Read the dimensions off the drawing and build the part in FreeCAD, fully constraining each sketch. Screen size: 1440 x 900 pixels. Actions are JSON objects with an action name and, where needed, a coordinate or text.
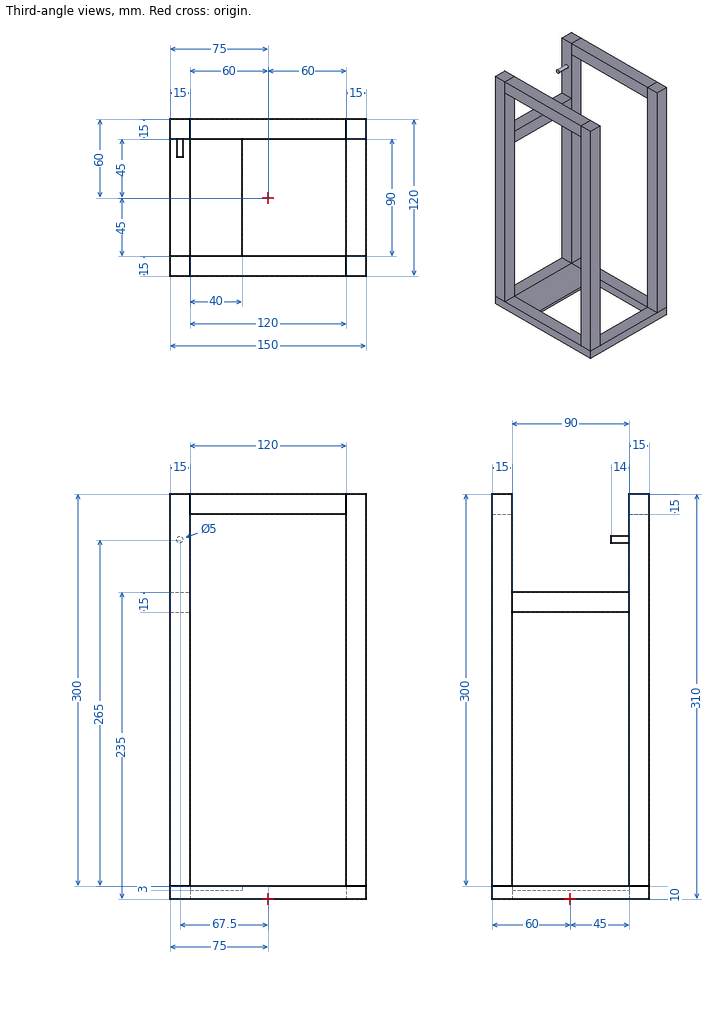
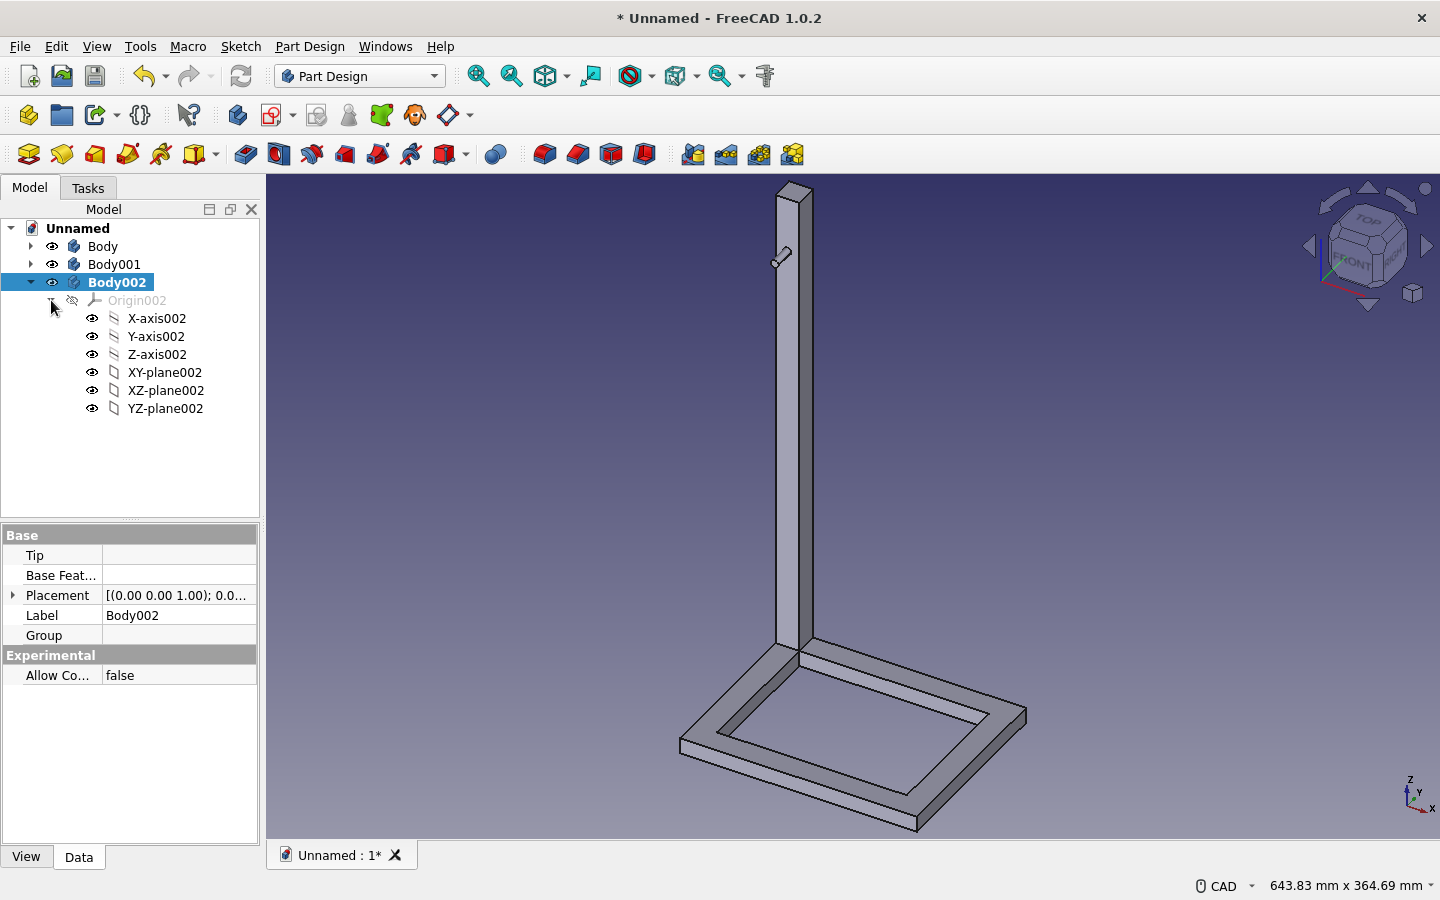
{"action": "left_click", "coordinate": [137, 372]}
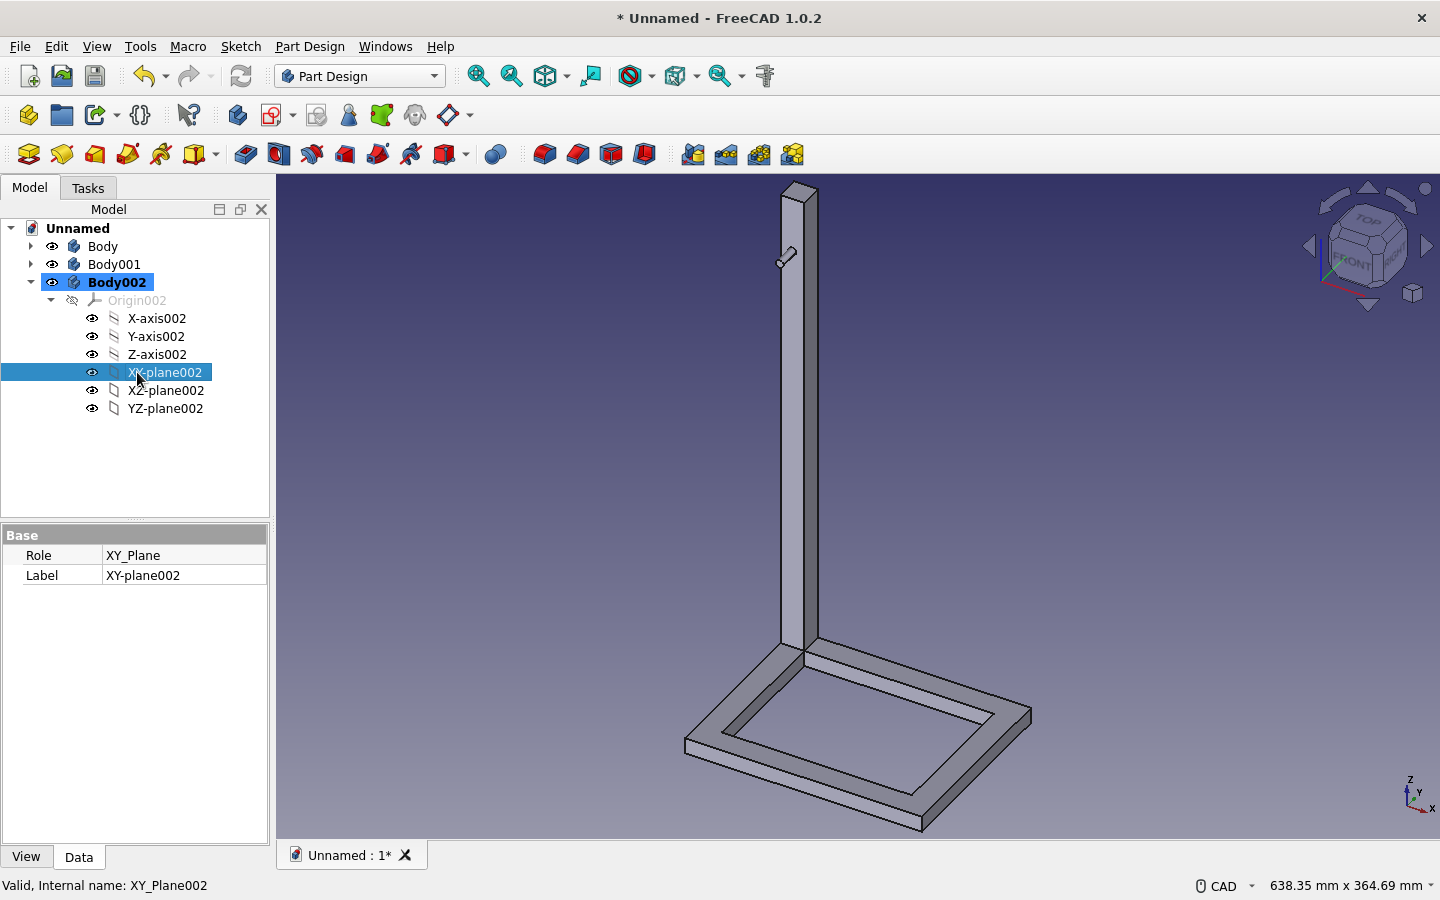
{"action": "left_click", "coordinate": [448, 116]}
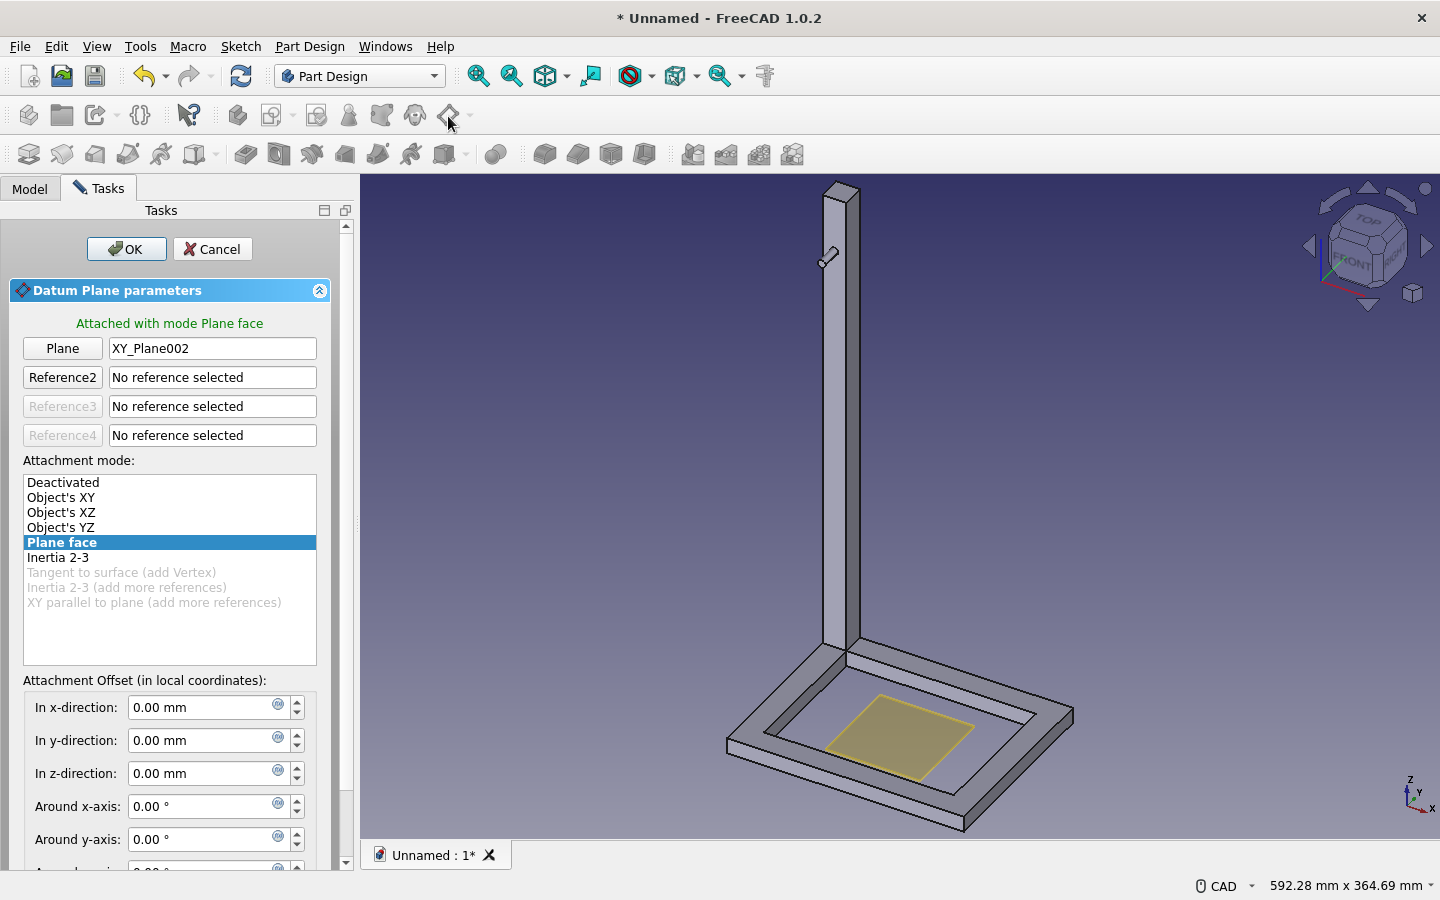
{"action": "triple_click", "coordinate": [210, 774]}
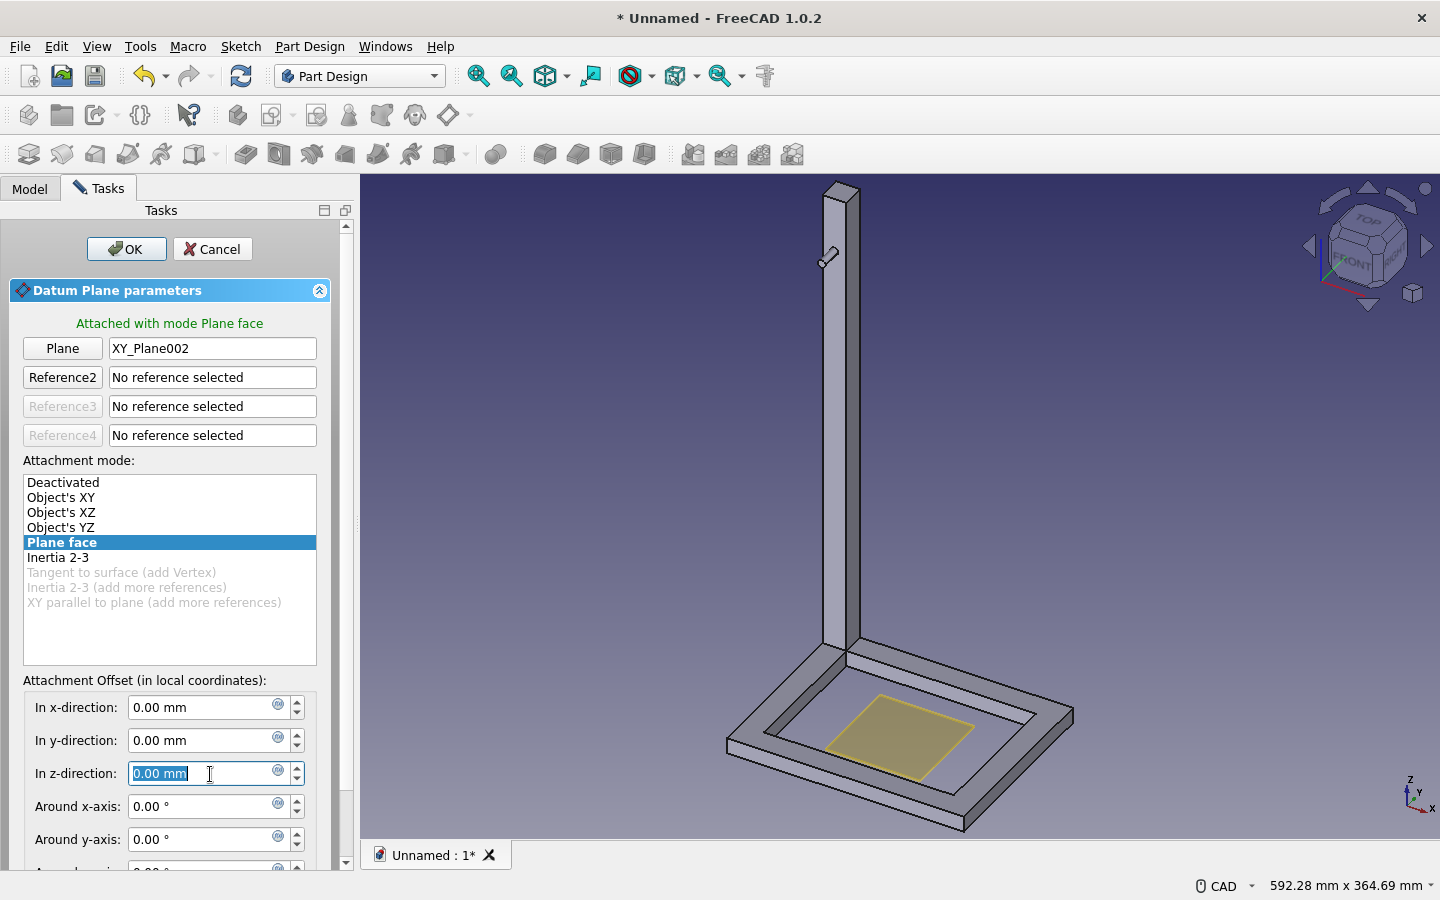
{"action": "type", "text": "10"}
{"action": "key", "text": "Tab"}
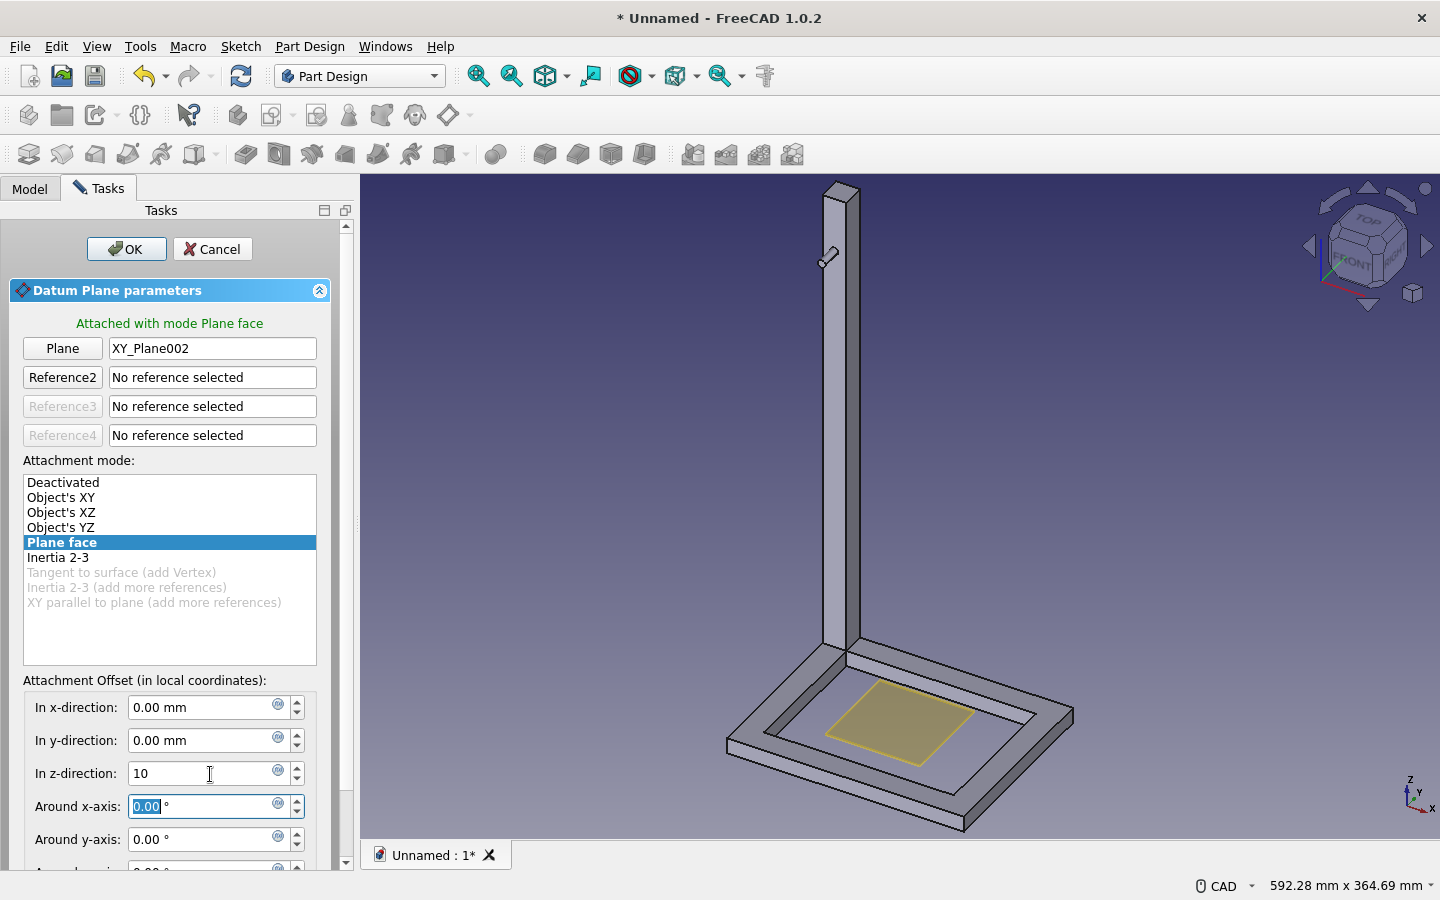
{"action": "left_click", "coordinate": [127, 249]}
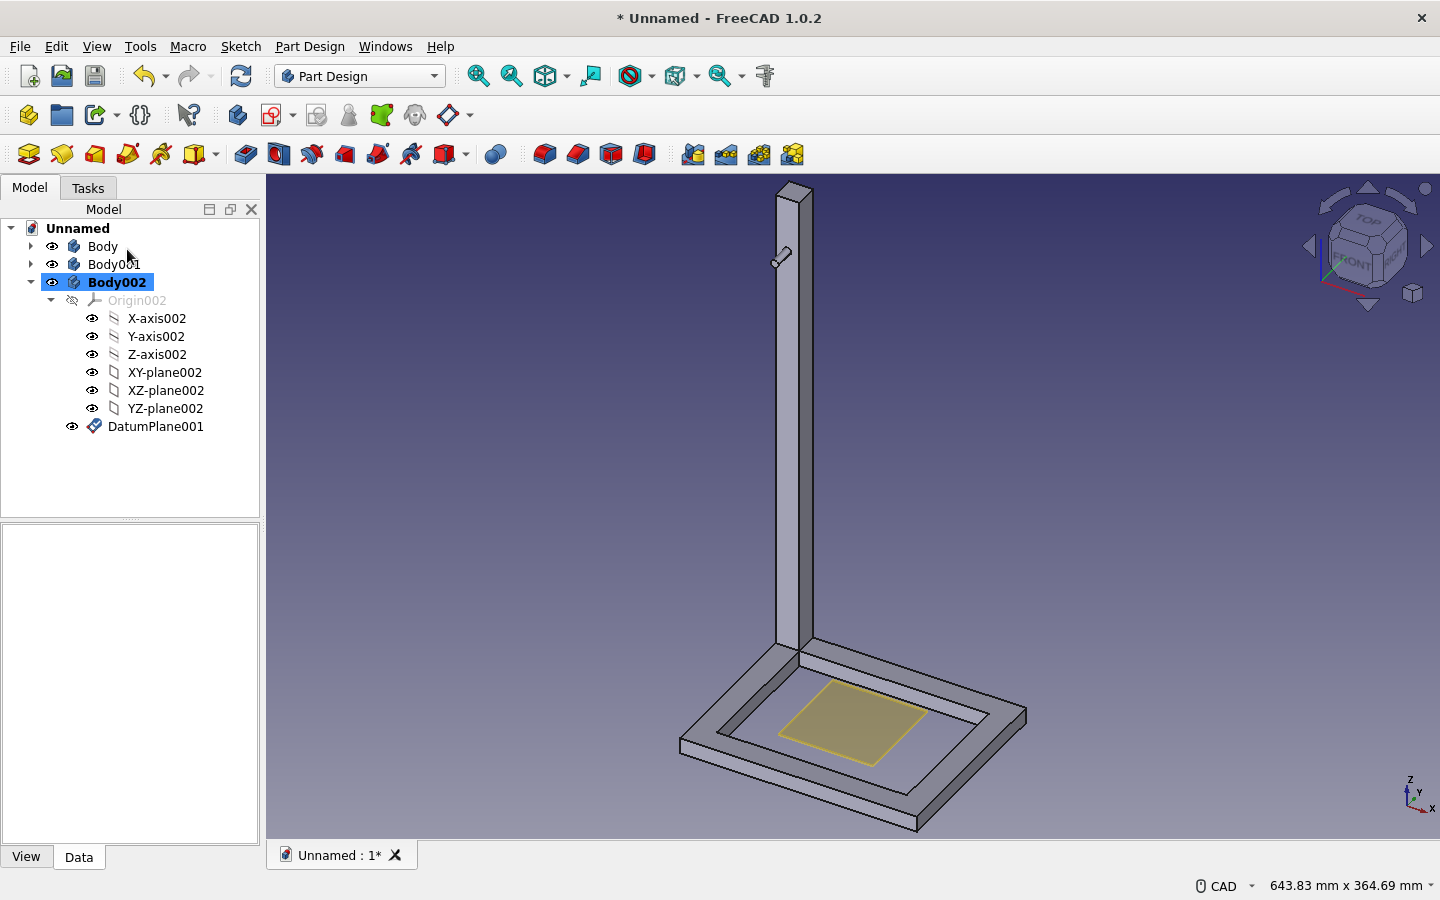
{"action": "left_click", "coordinate": [117, 426]}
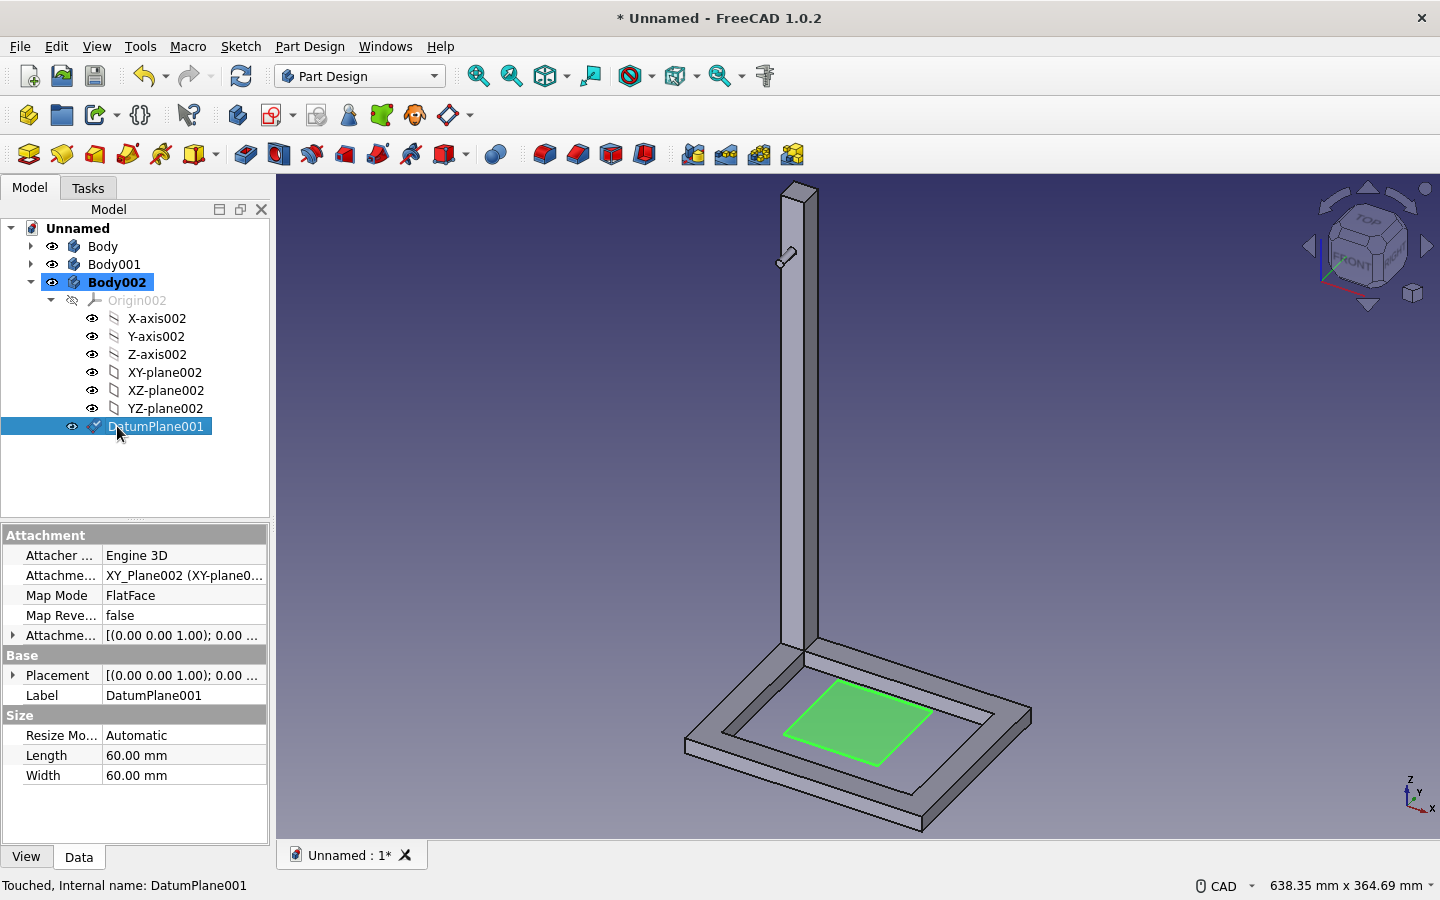
{"action": "left_click", "coordinate": [270, 116]}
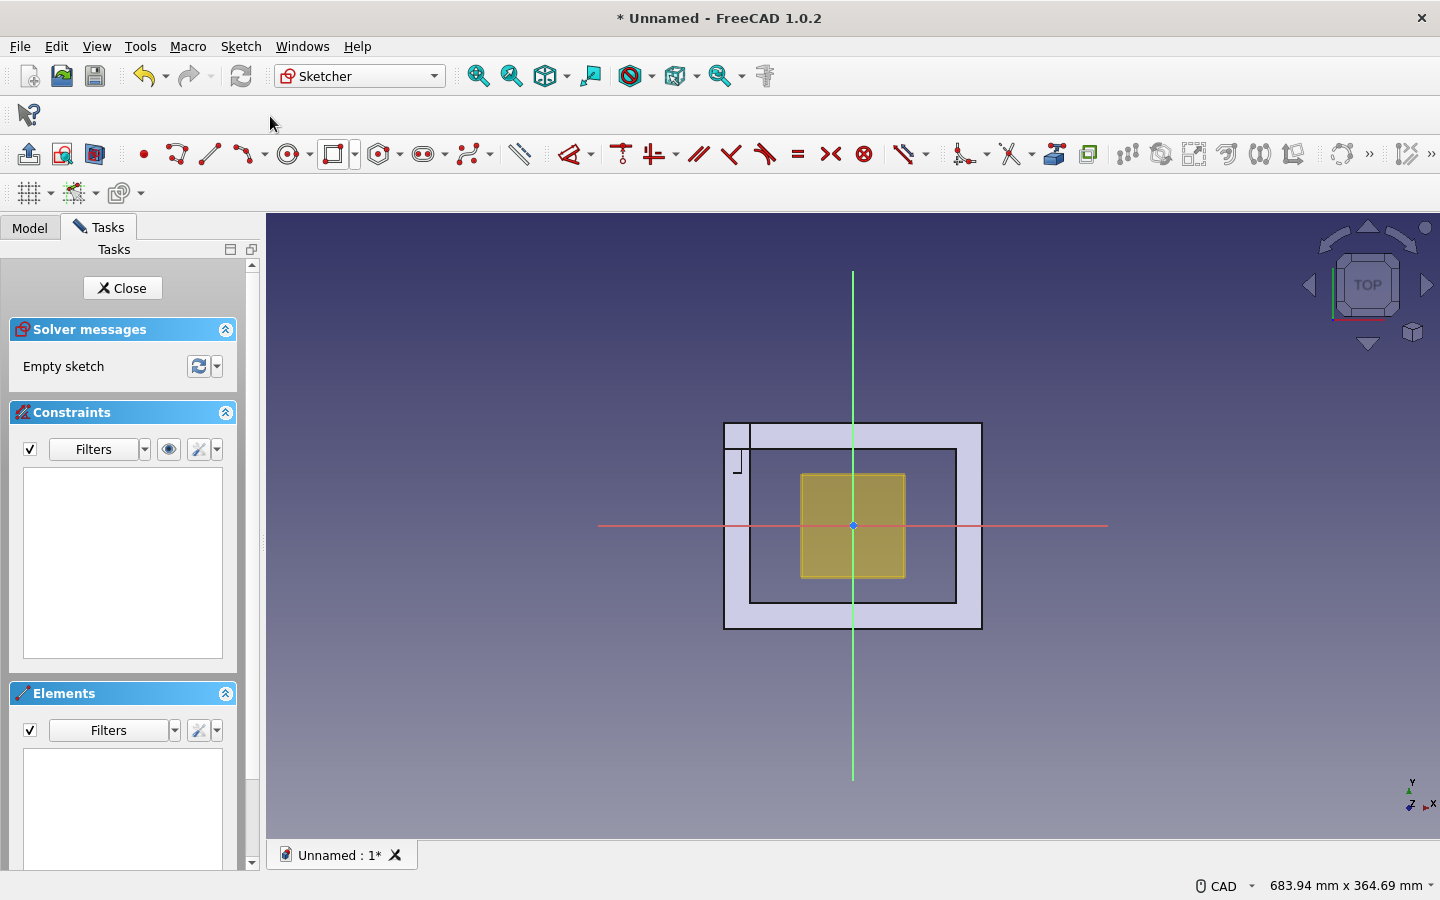
{"action": "scroll", "coordinate": [734, 622], "scroll_direction": "up", "scroll_amount": 14}